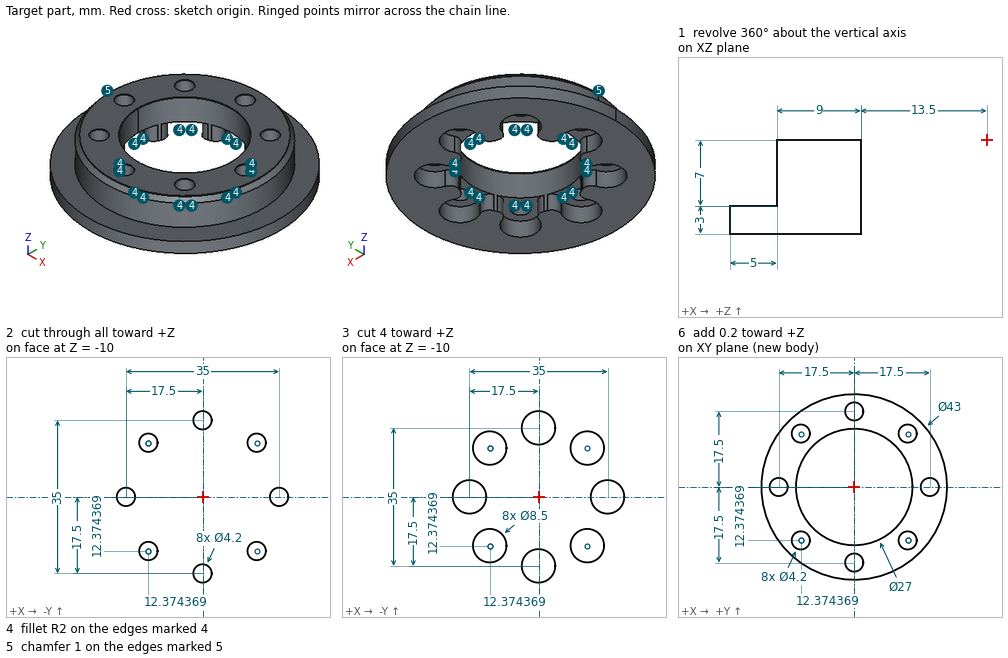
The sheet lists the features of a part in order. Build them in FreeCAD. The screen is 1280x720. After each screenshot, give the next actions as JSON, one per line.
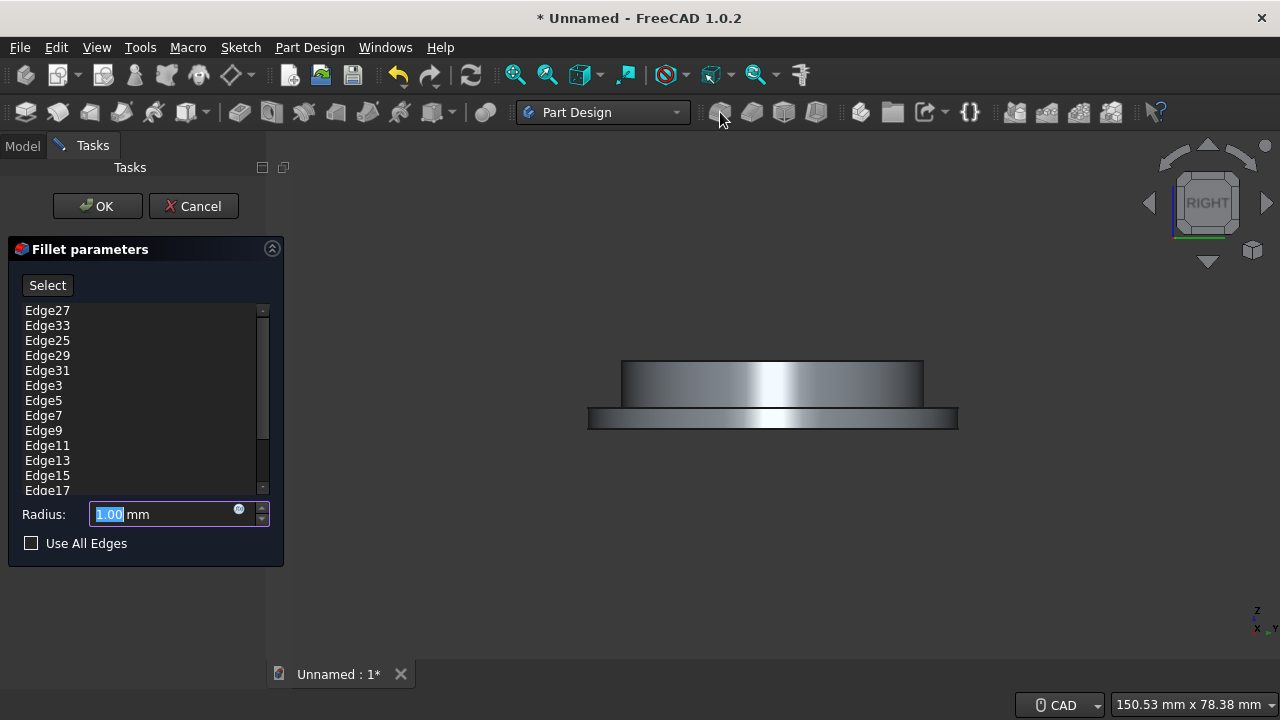
{"action": "type", "text": "2"}
{"action": "key", "text": "Tab"}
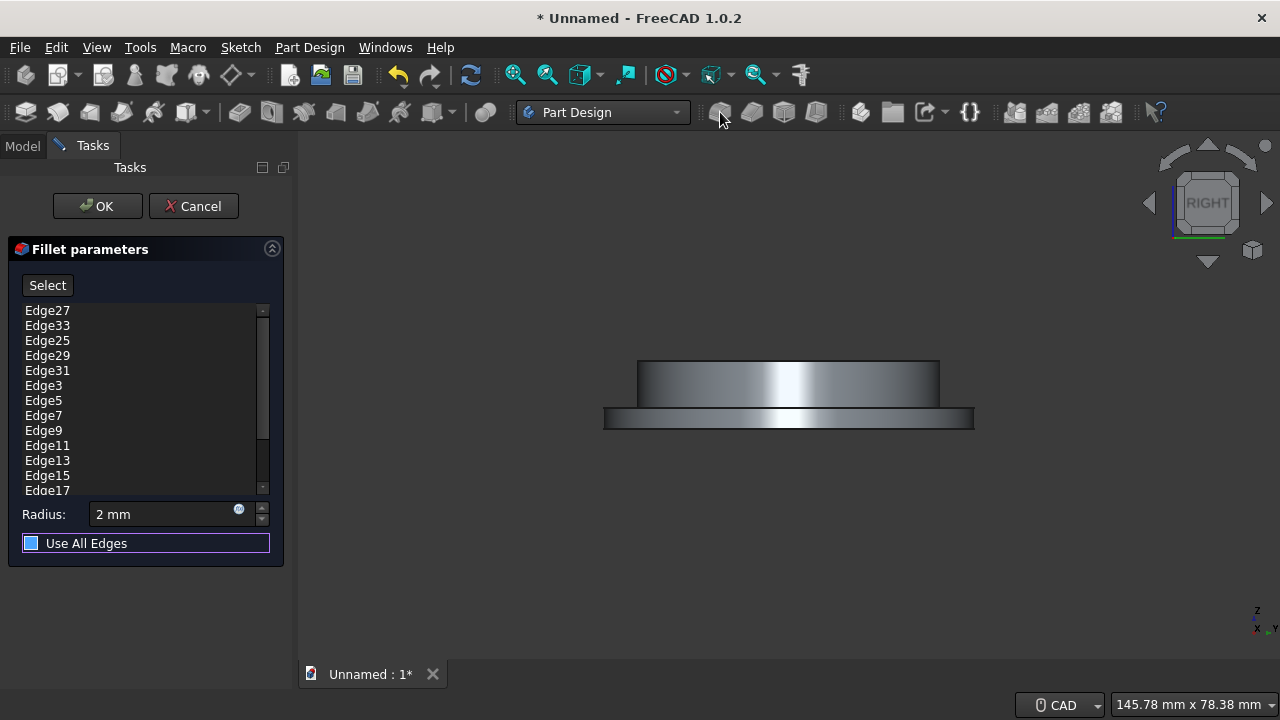
{"action": "left_click", "coordinate": [98, 206]}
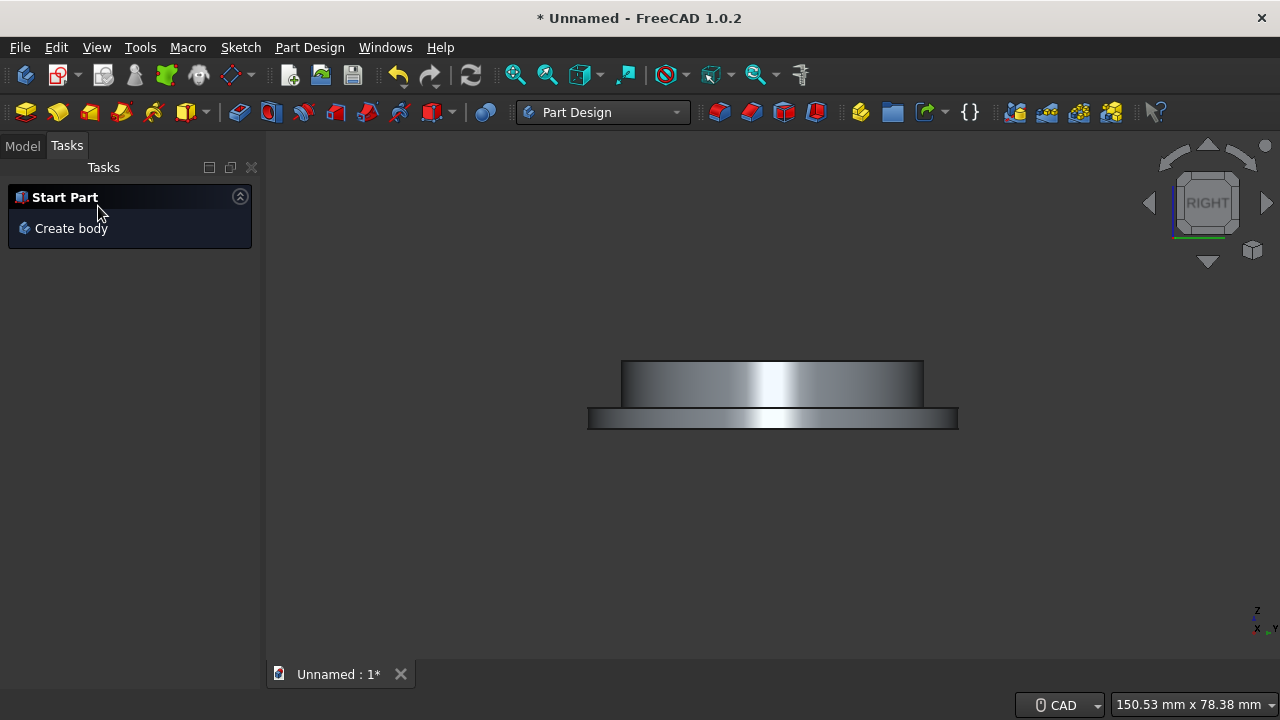
{"action": "key", "text": "v f"}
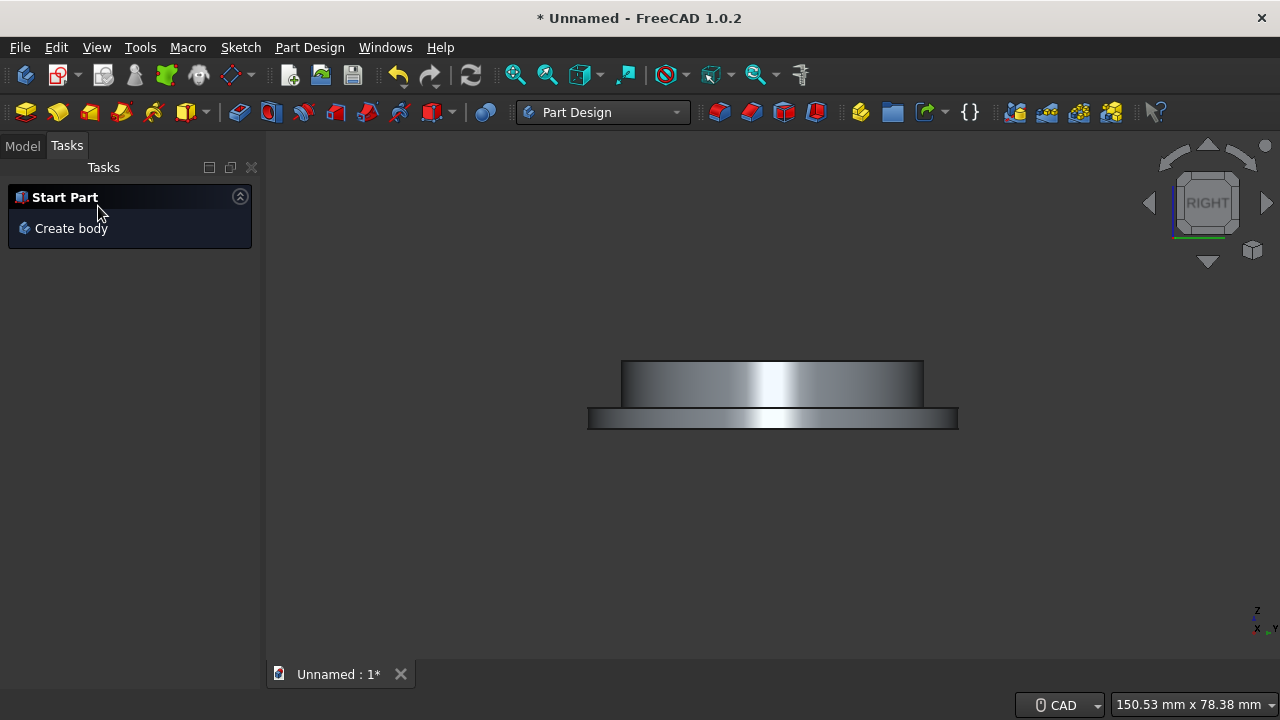
{"action": "left_click", "coordinate": [773, 360]}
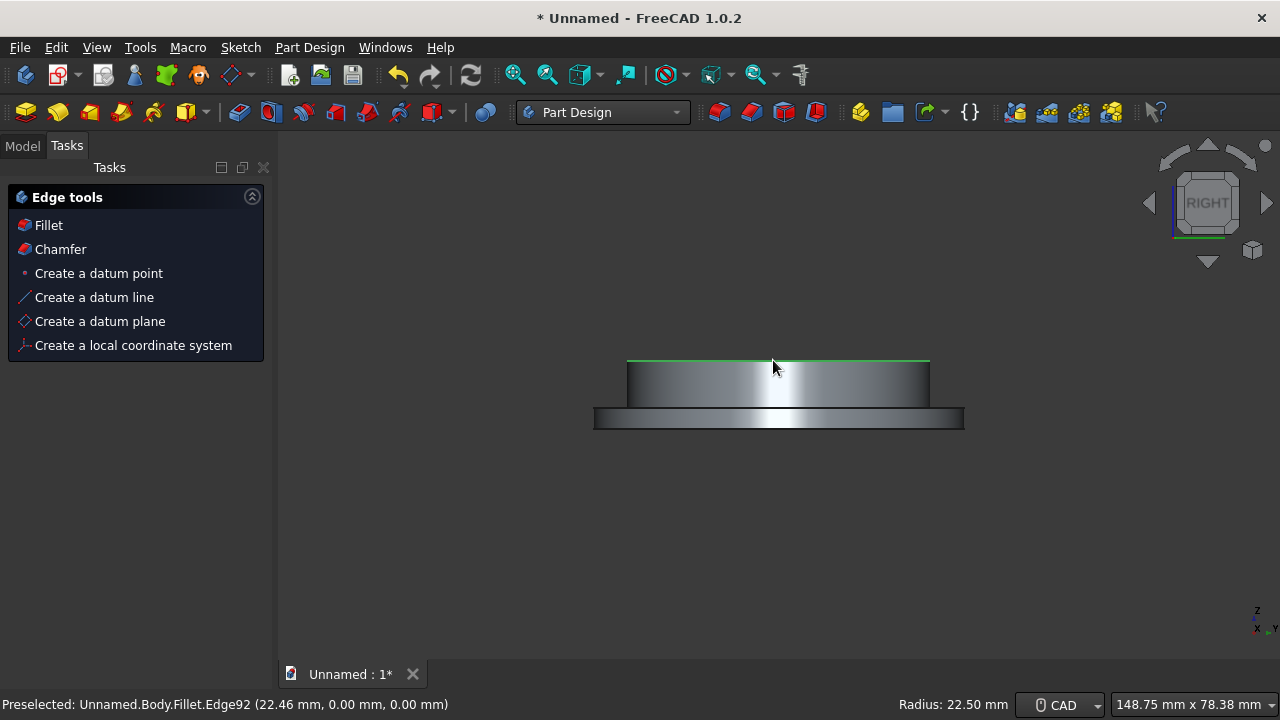
{"action": "left_click", "coordinate": [752, 112]}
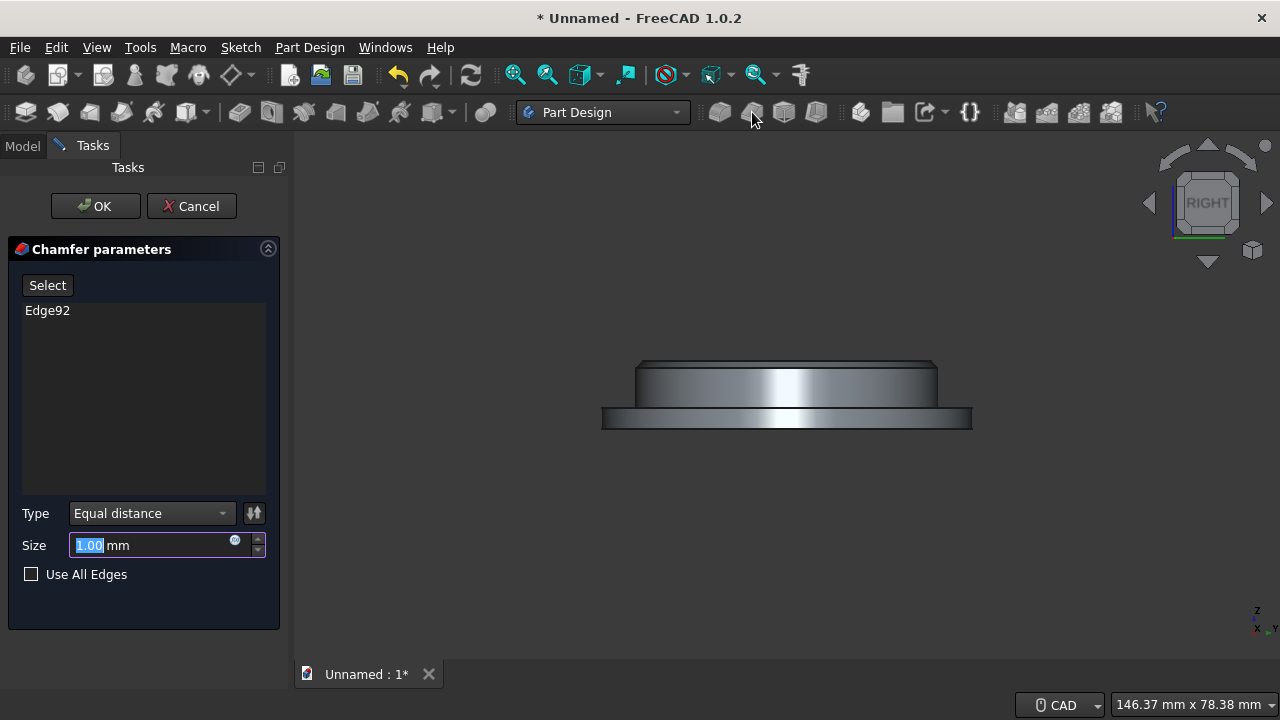
{"action": "type", "text": "1"}
{"action": "key", "text": "Tab"}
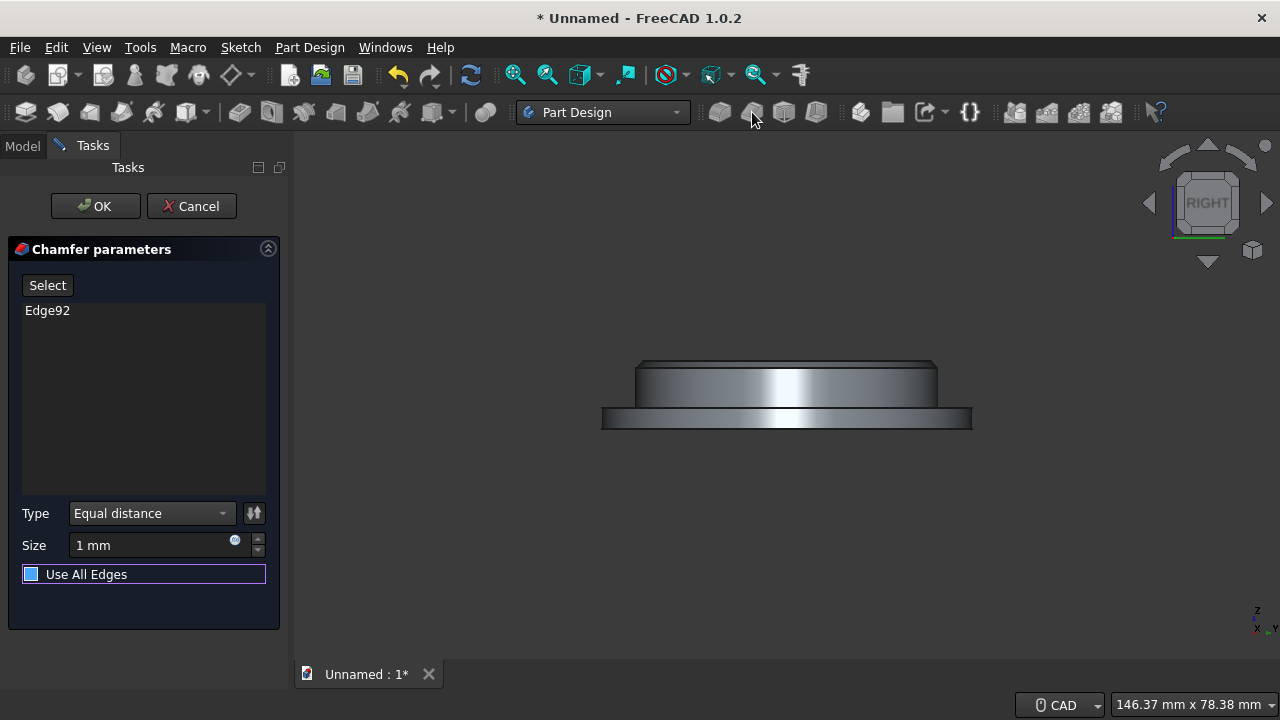
{"action": "left_click", "coordinate": [96, 206]}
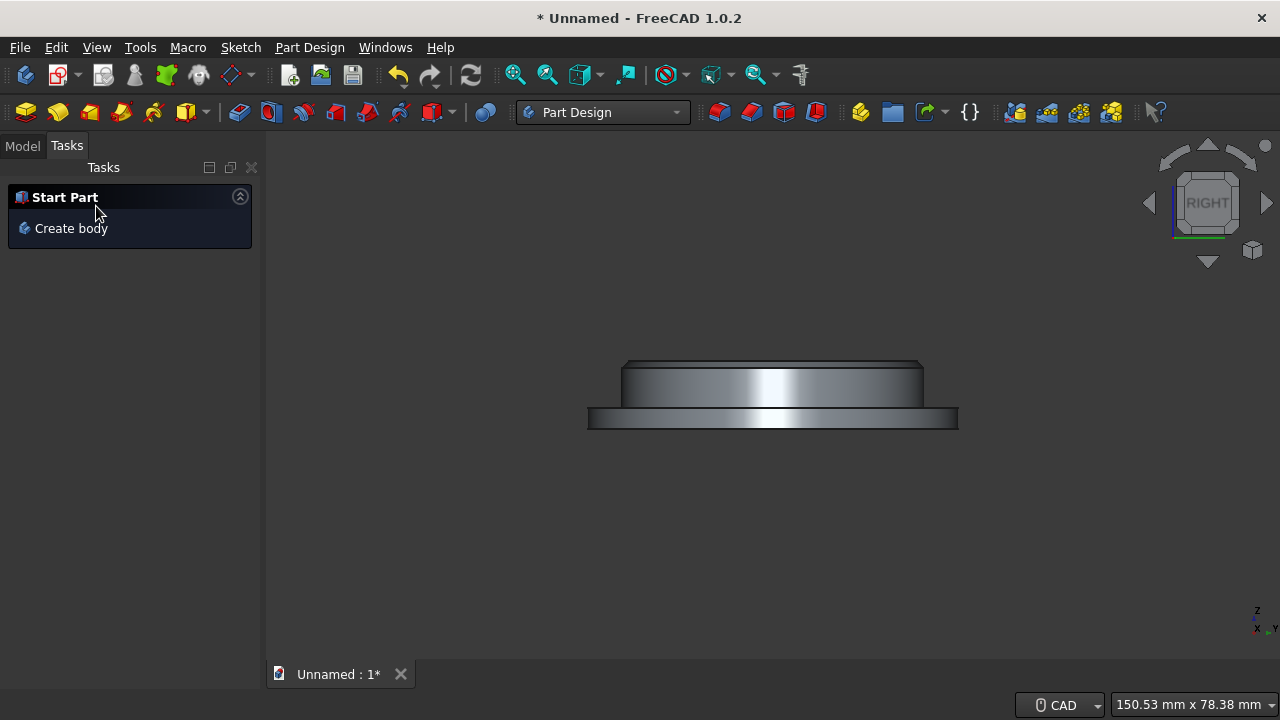
{"action": "left_click", "coordinate": [516, 76]}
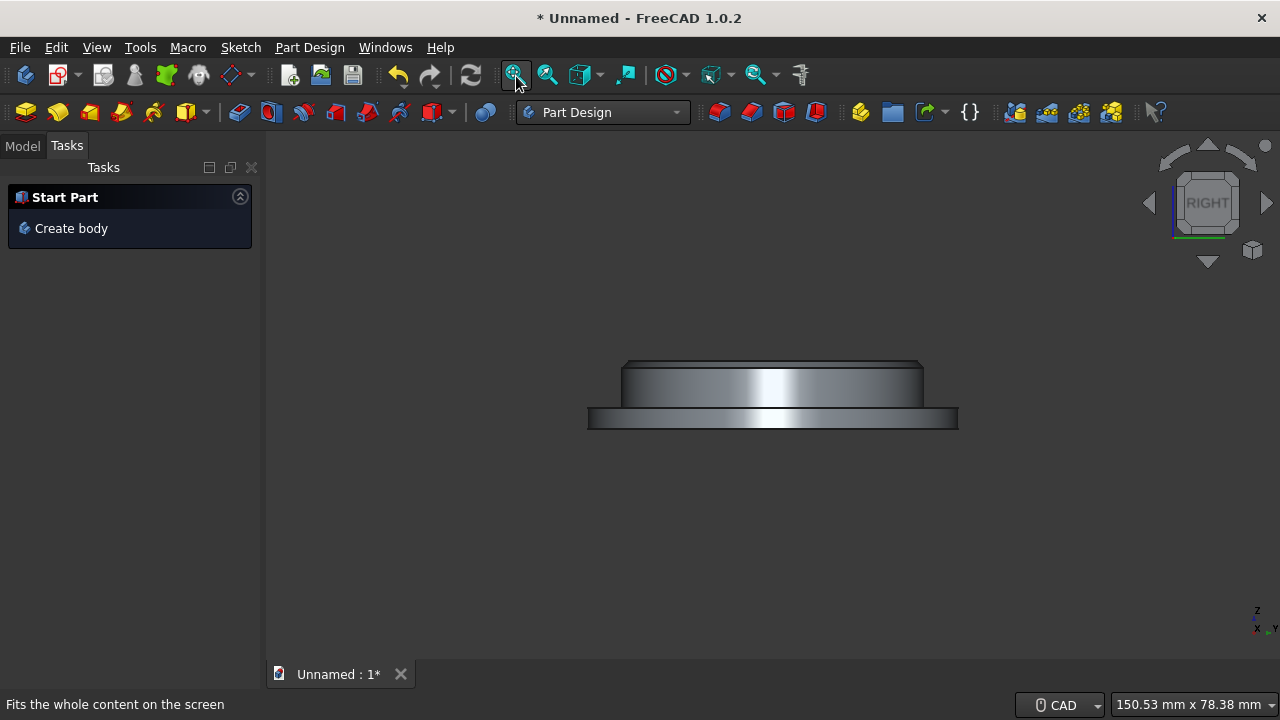
{"action": "left_click", "coordinate": [26, 76]}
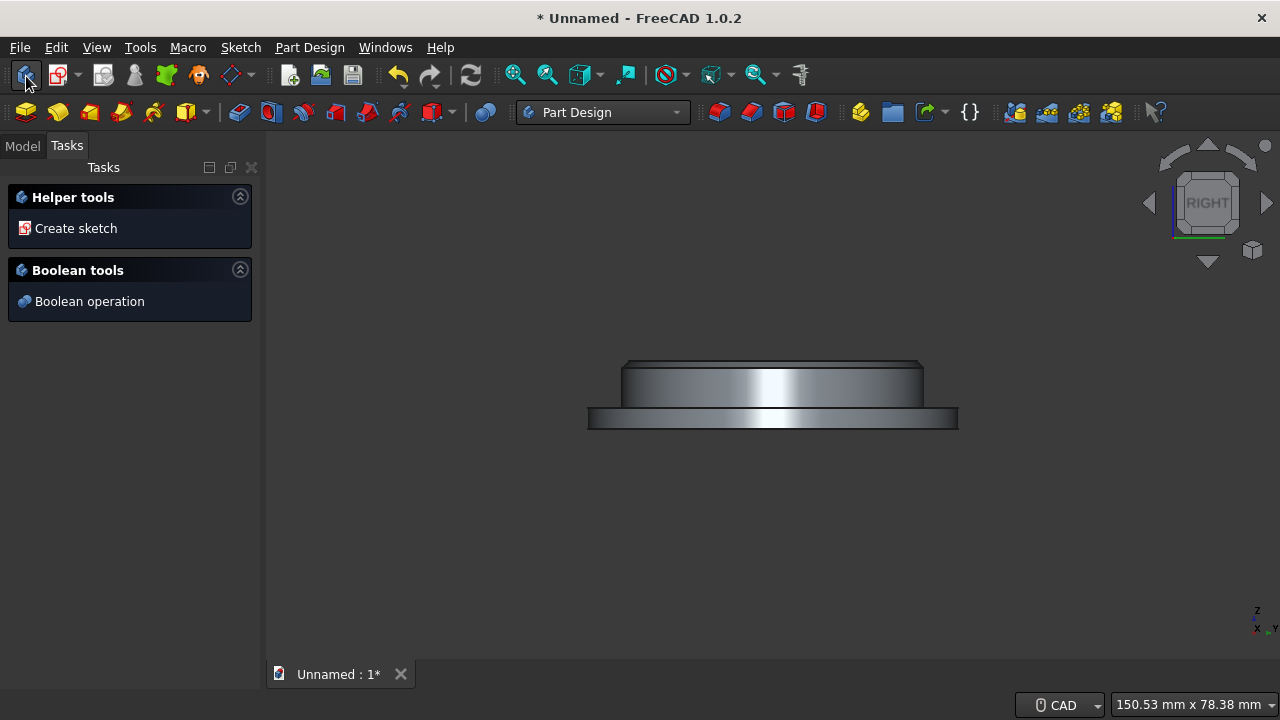
{"action": "left_click", "coordinate": [306, 619]}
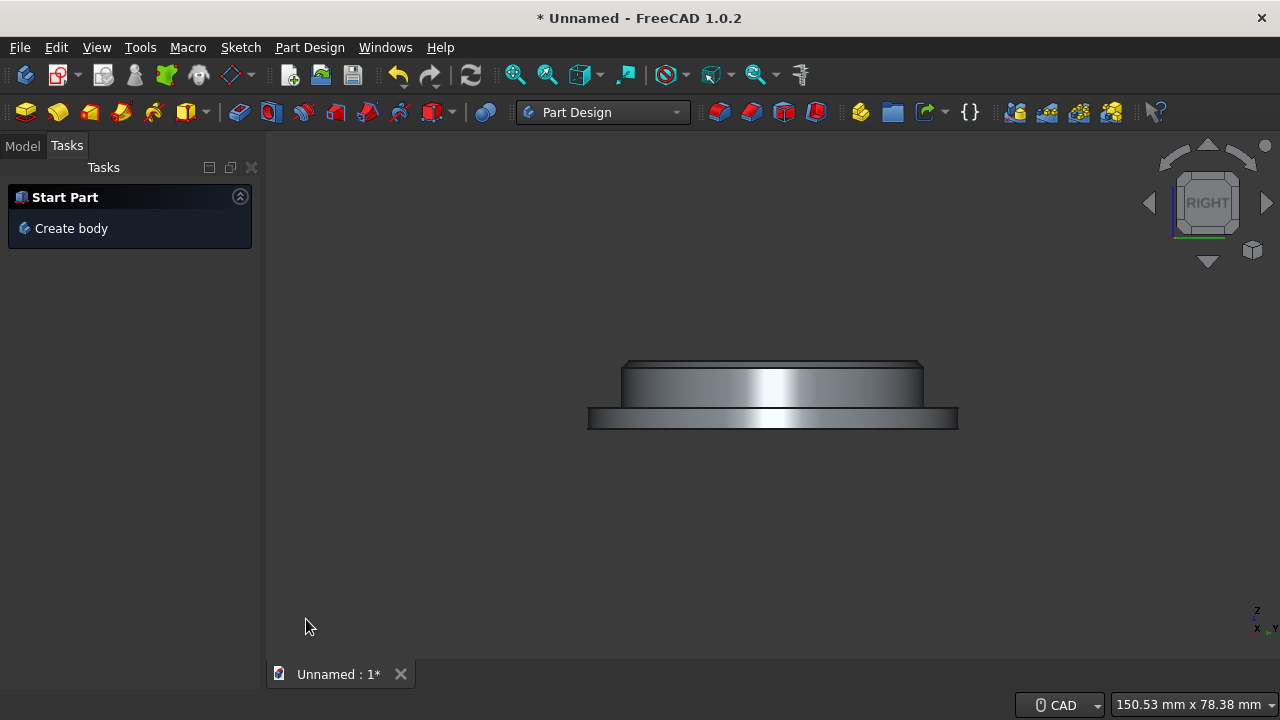
{"action": "left_click", "coordinate": [58, 76]}